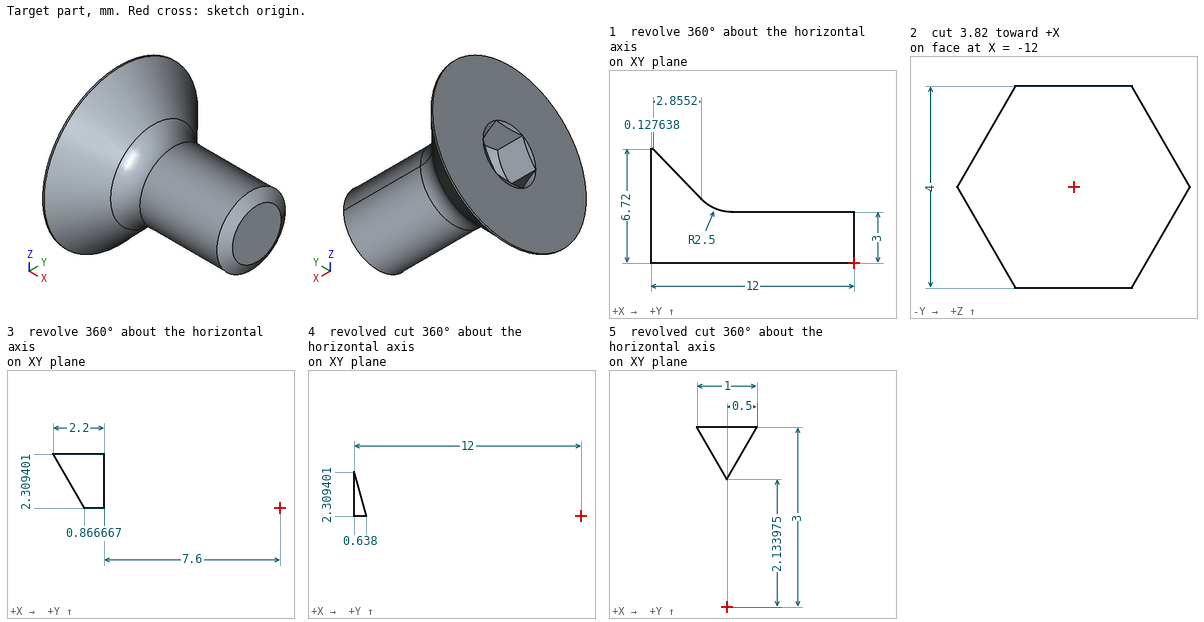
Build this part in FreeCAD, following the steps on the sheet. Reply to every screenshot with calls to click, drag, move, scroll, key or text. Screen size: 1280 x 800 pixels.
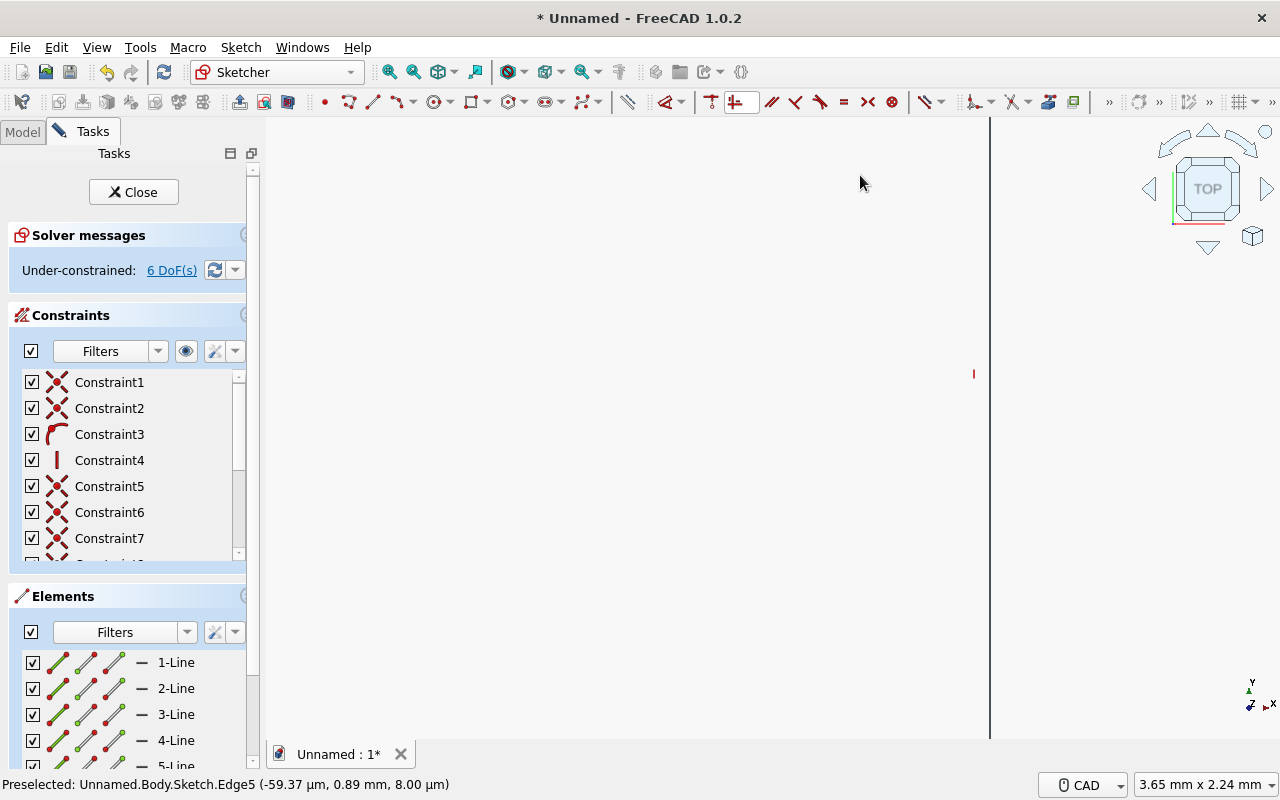
key(d)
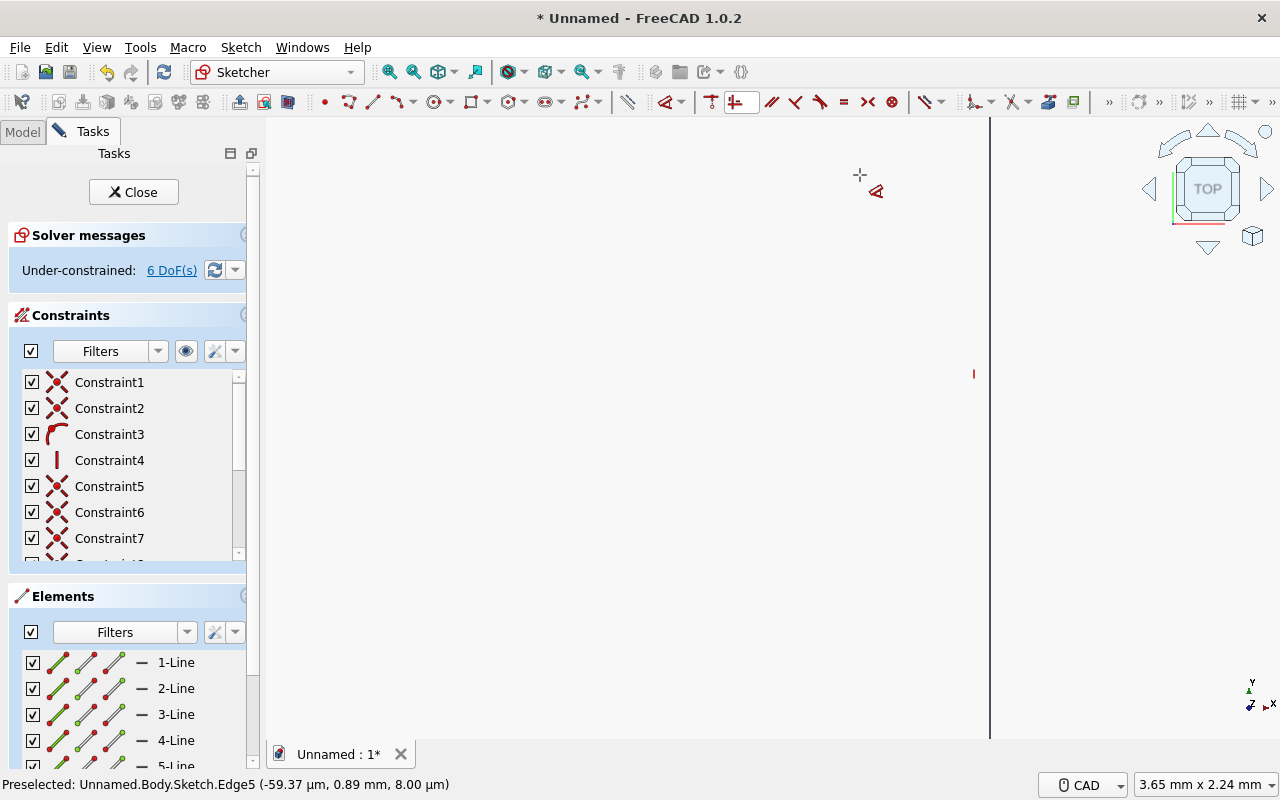
scroll(978, 541, down, 9)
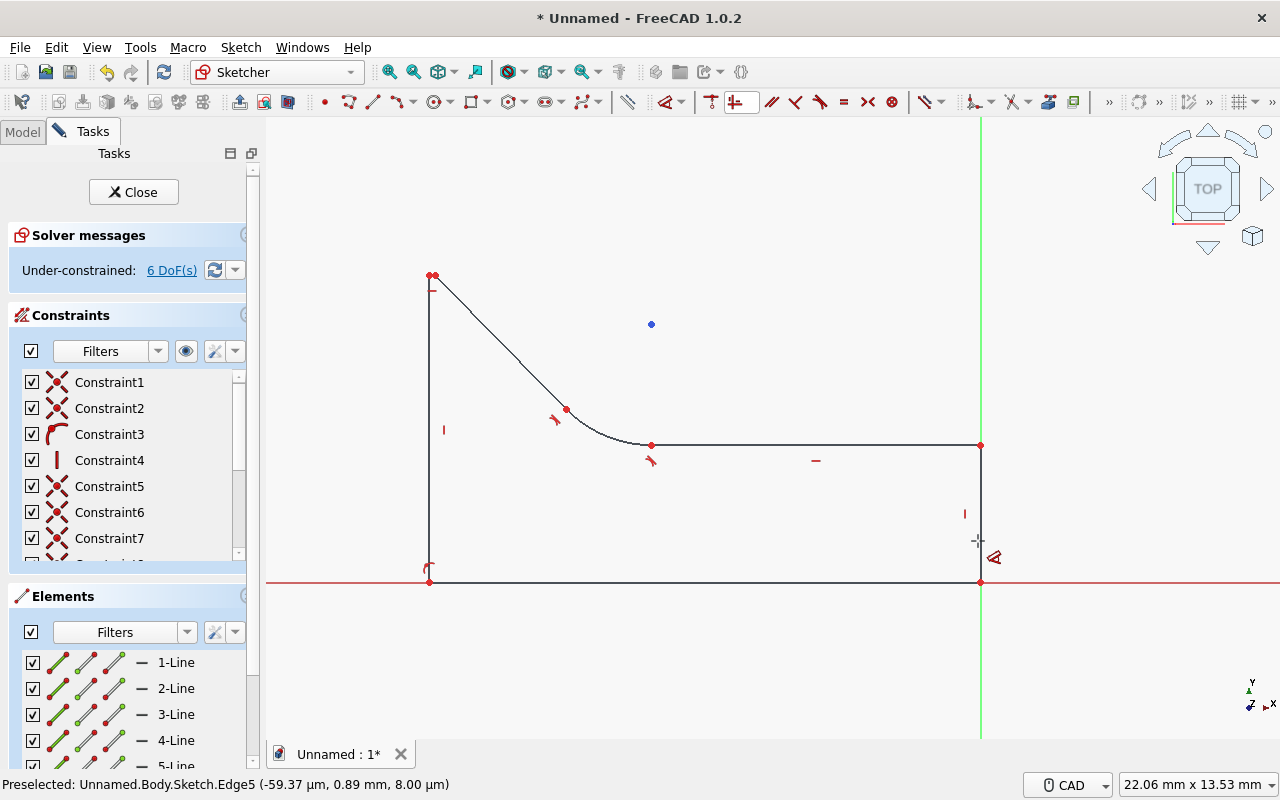
click(588, 427)
click(571, 454)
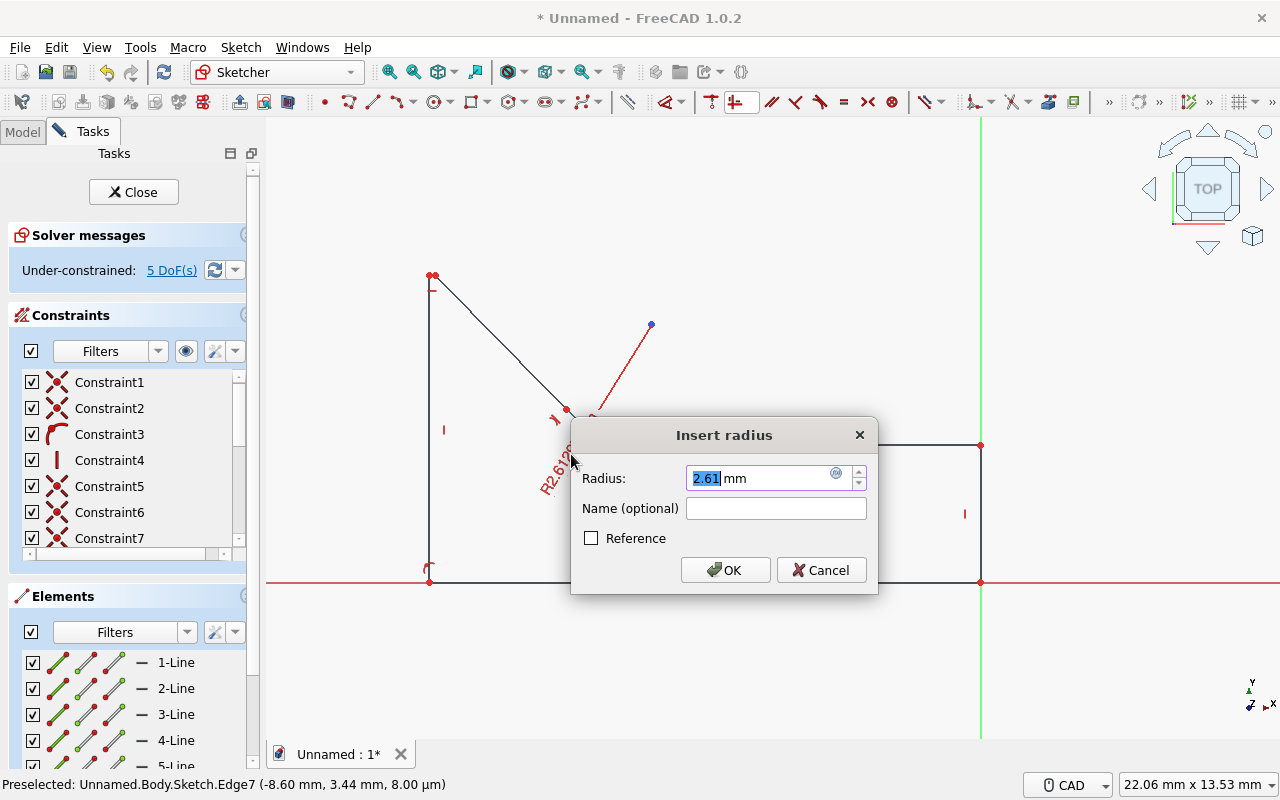
text(2.5)
key(Return)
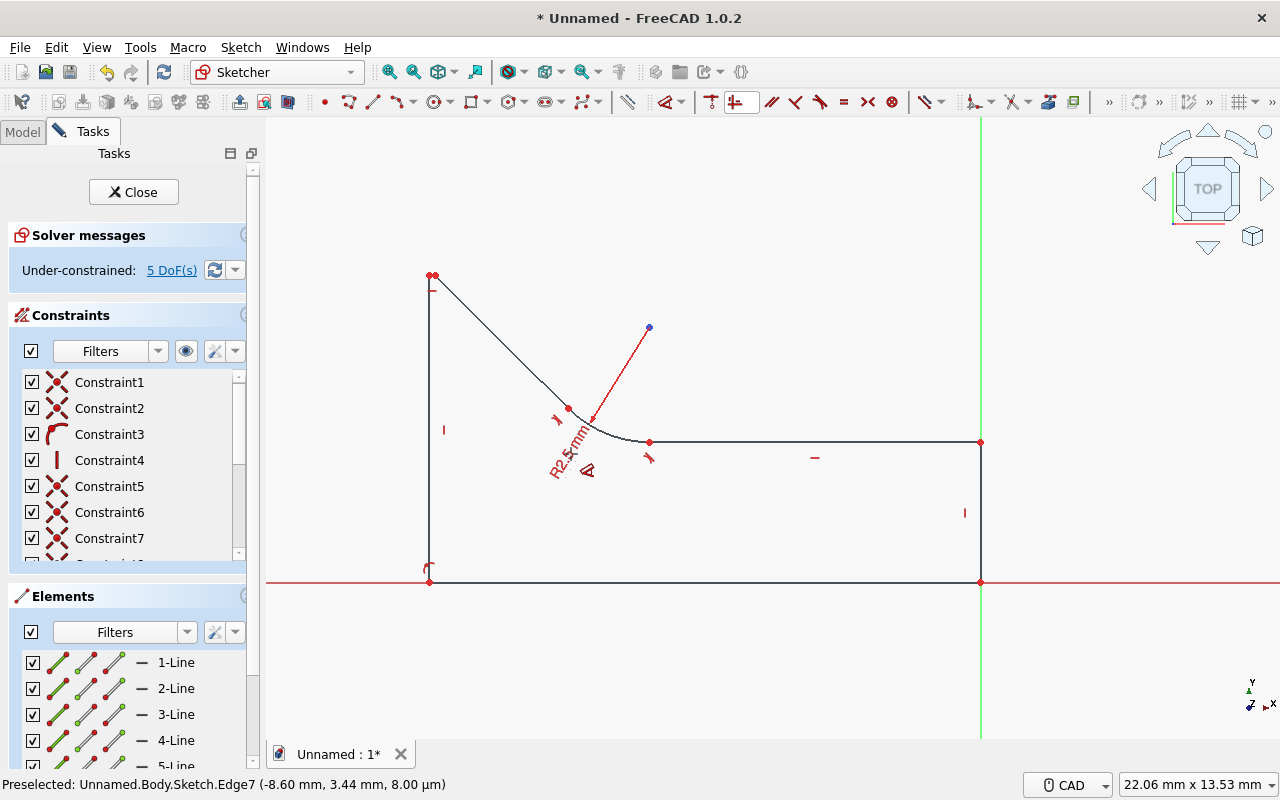
click(981, 541)
click(1015, 512)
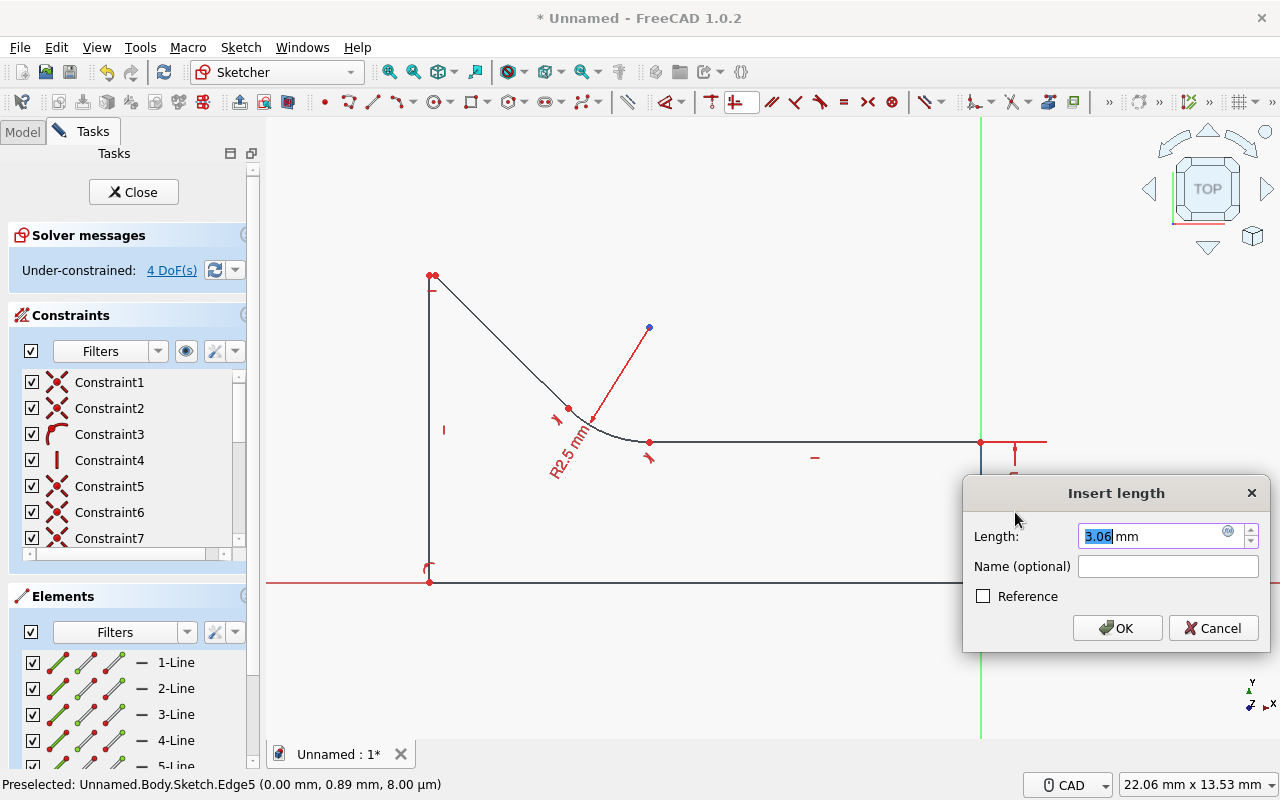
text(3)
key(Return)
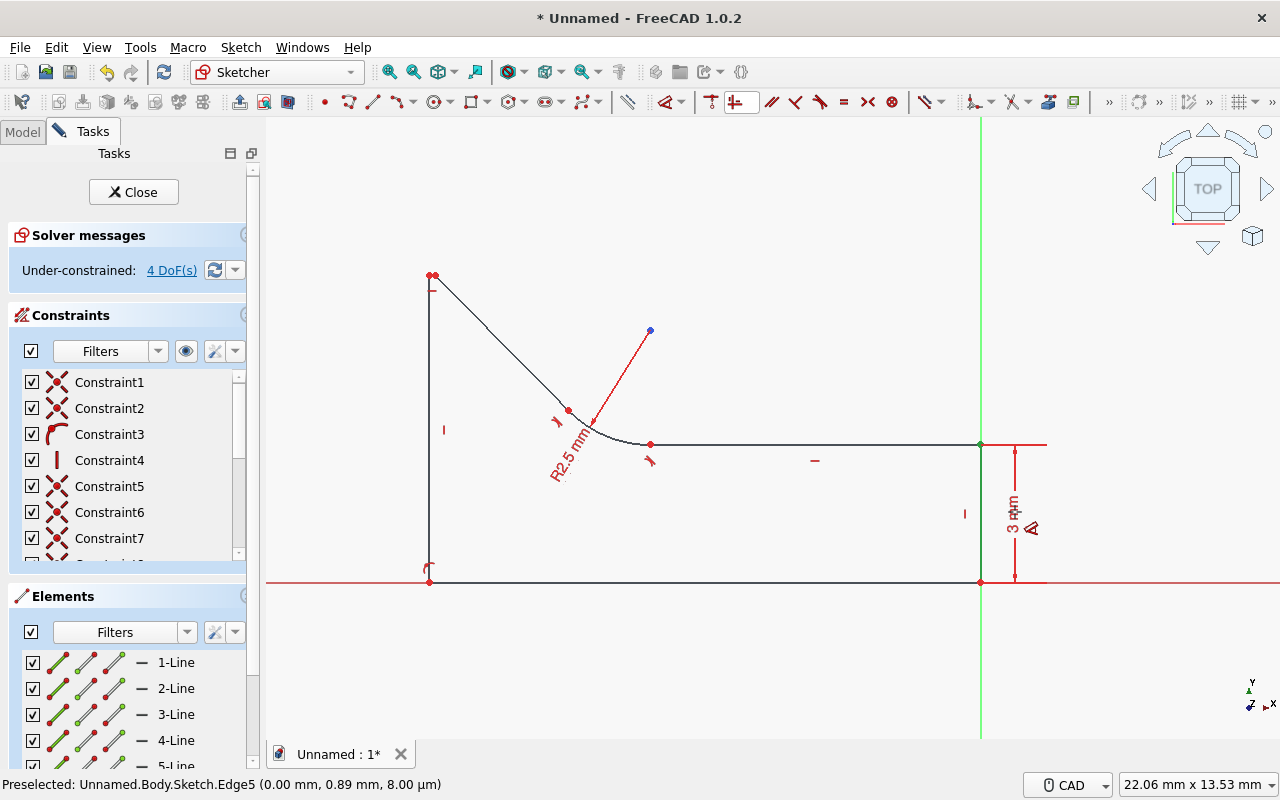
click(595, 583)
click(705, 617)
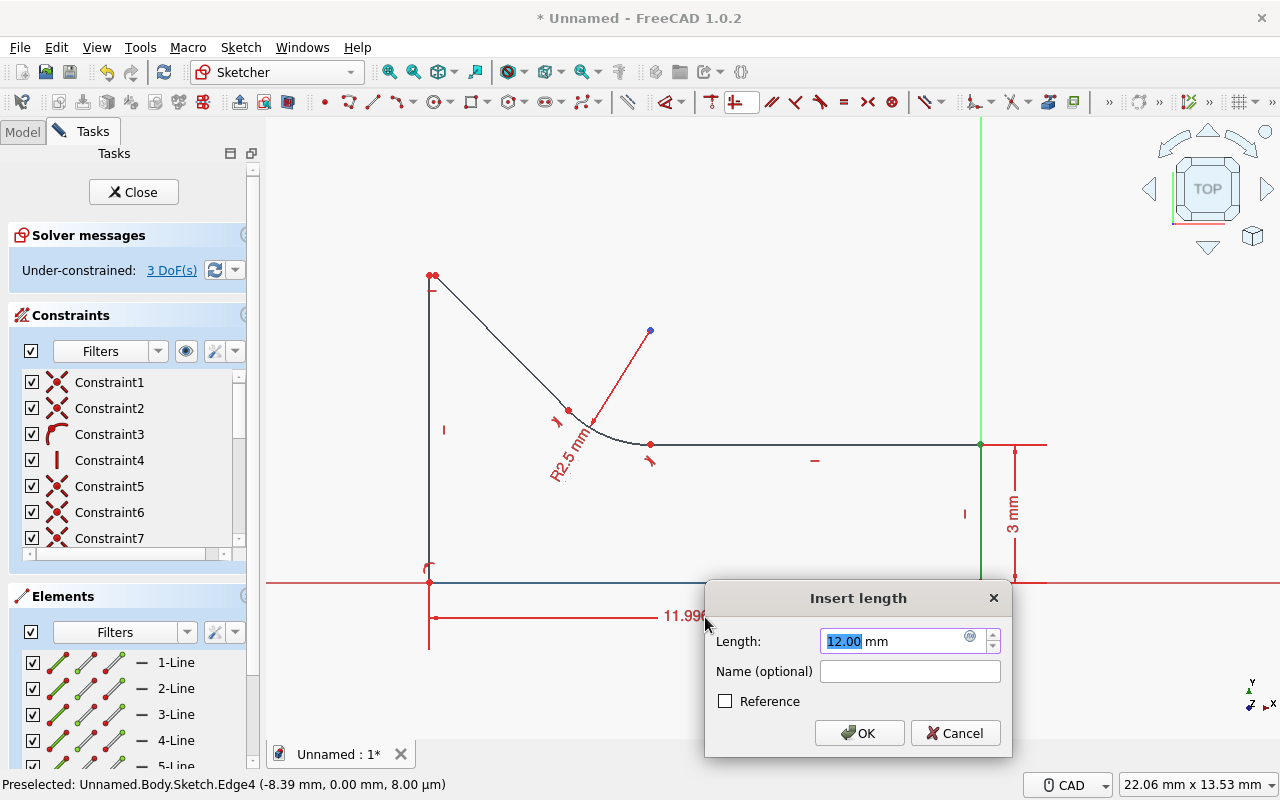
text(12)
key(Return)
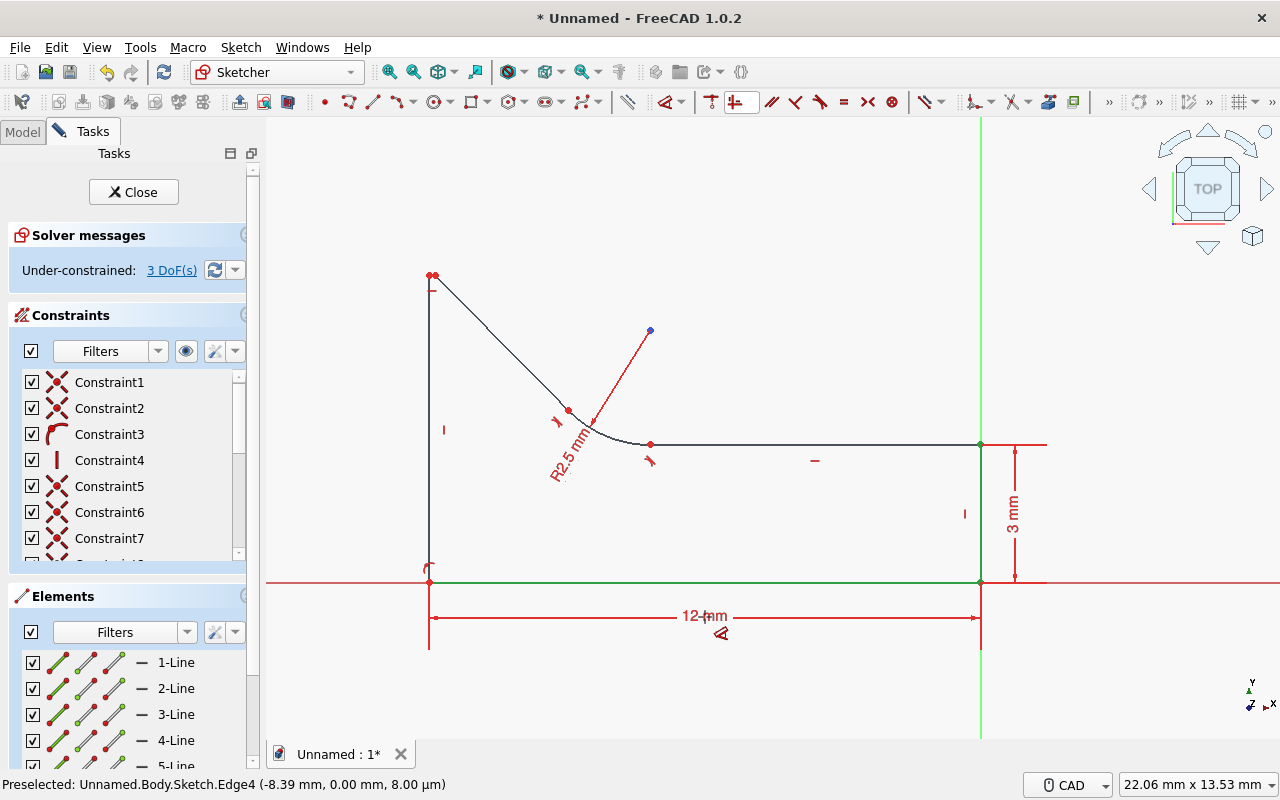
click(429, 368)
click(395, 429)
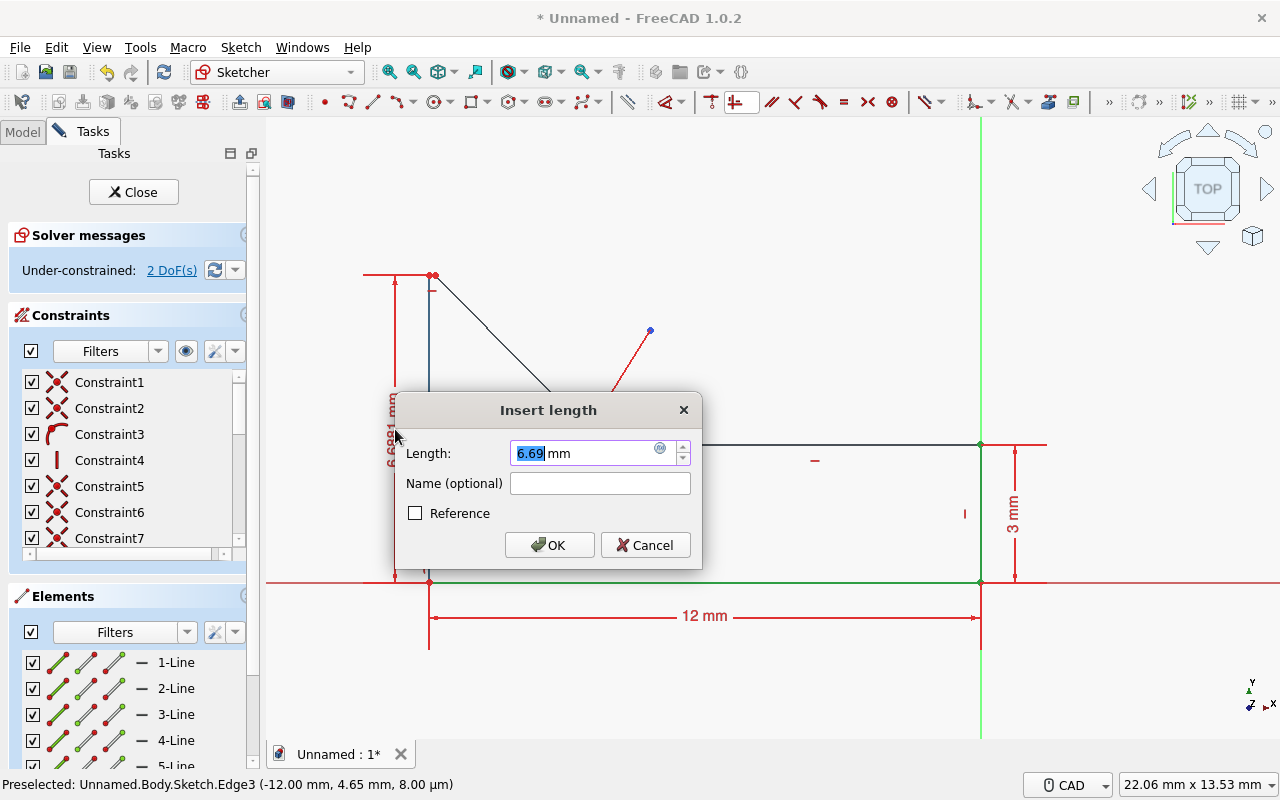
text(6.72)
key(Return)